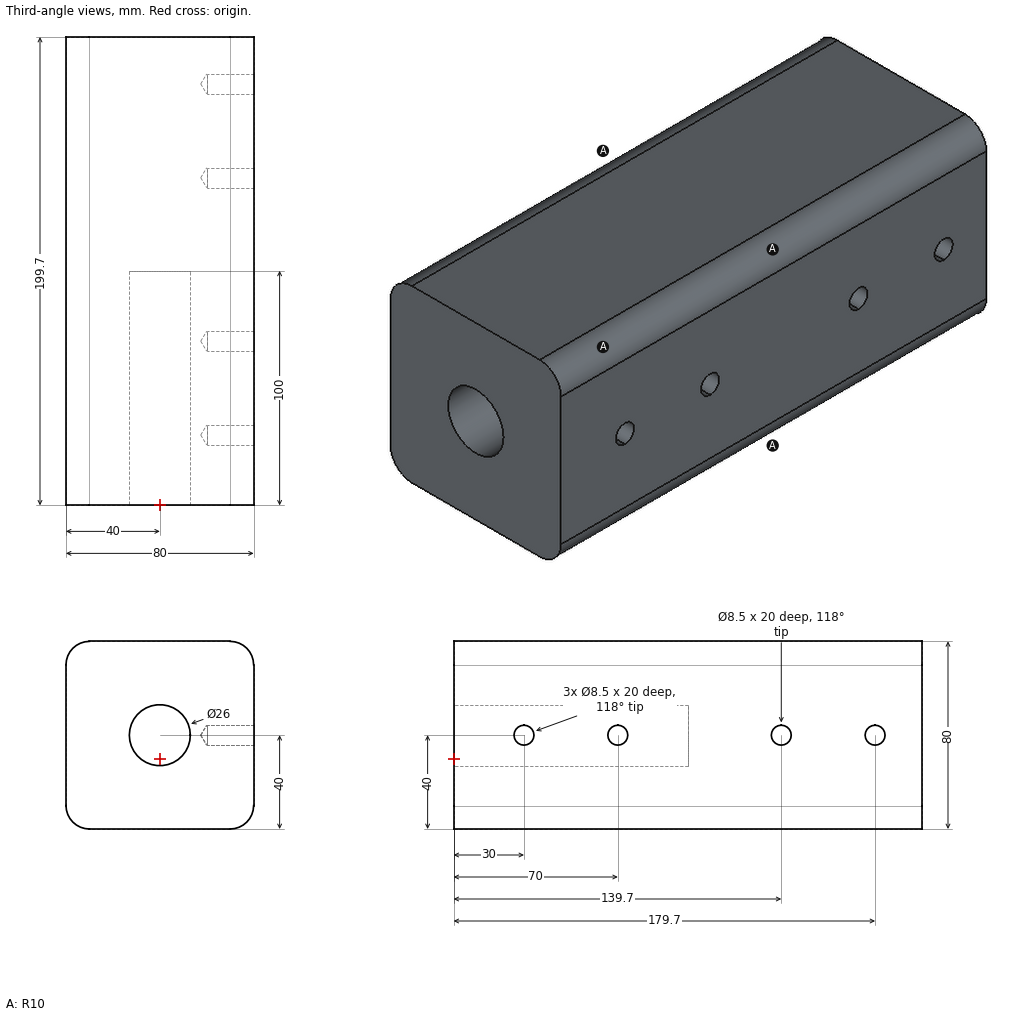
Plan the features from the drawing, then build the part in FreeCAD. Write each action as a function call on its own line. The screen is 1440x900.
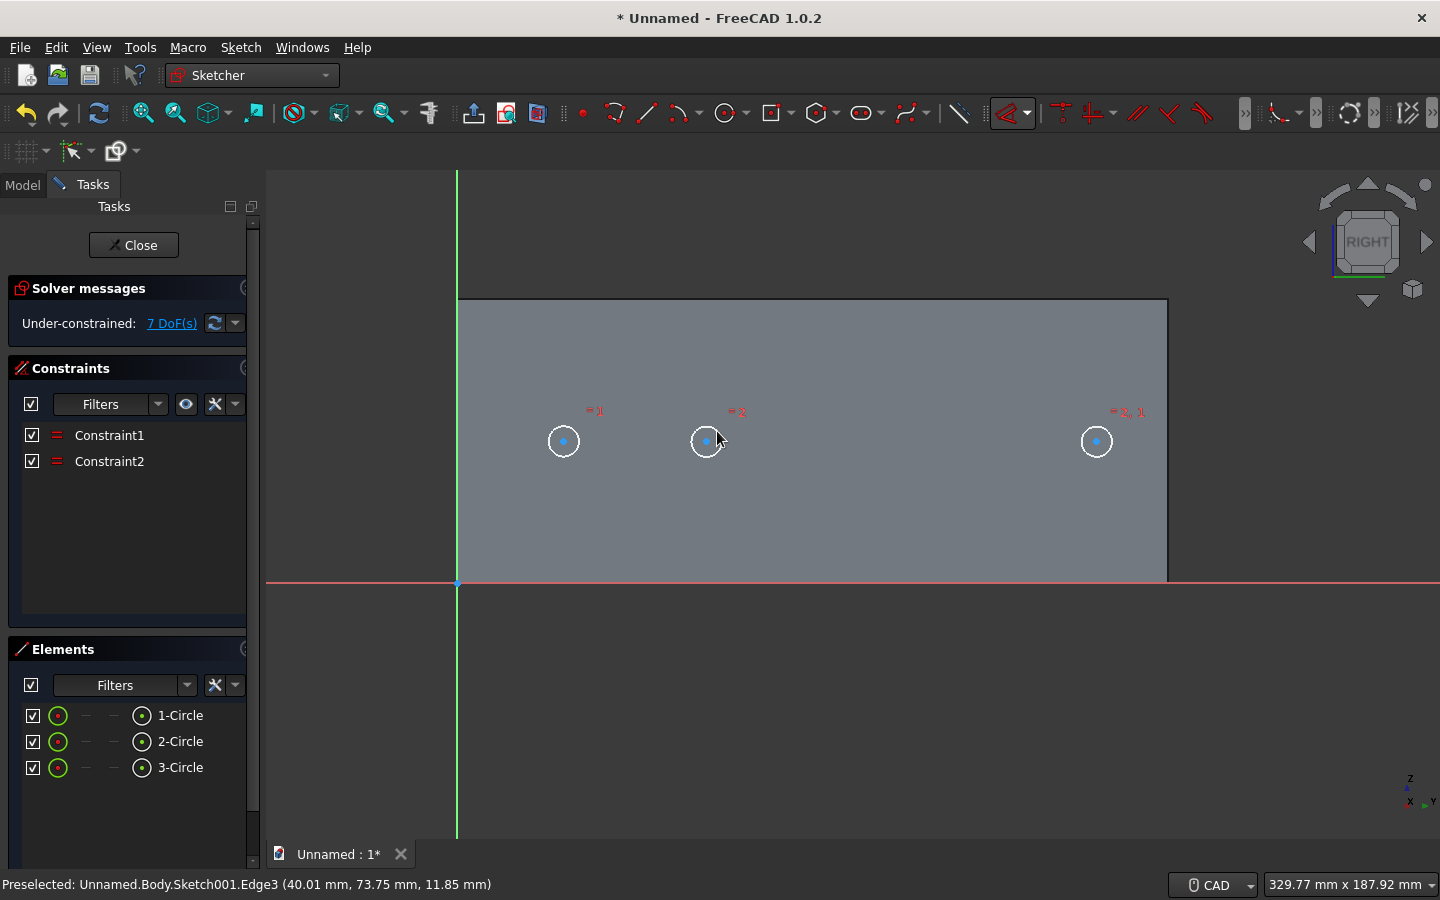
click(564, 441)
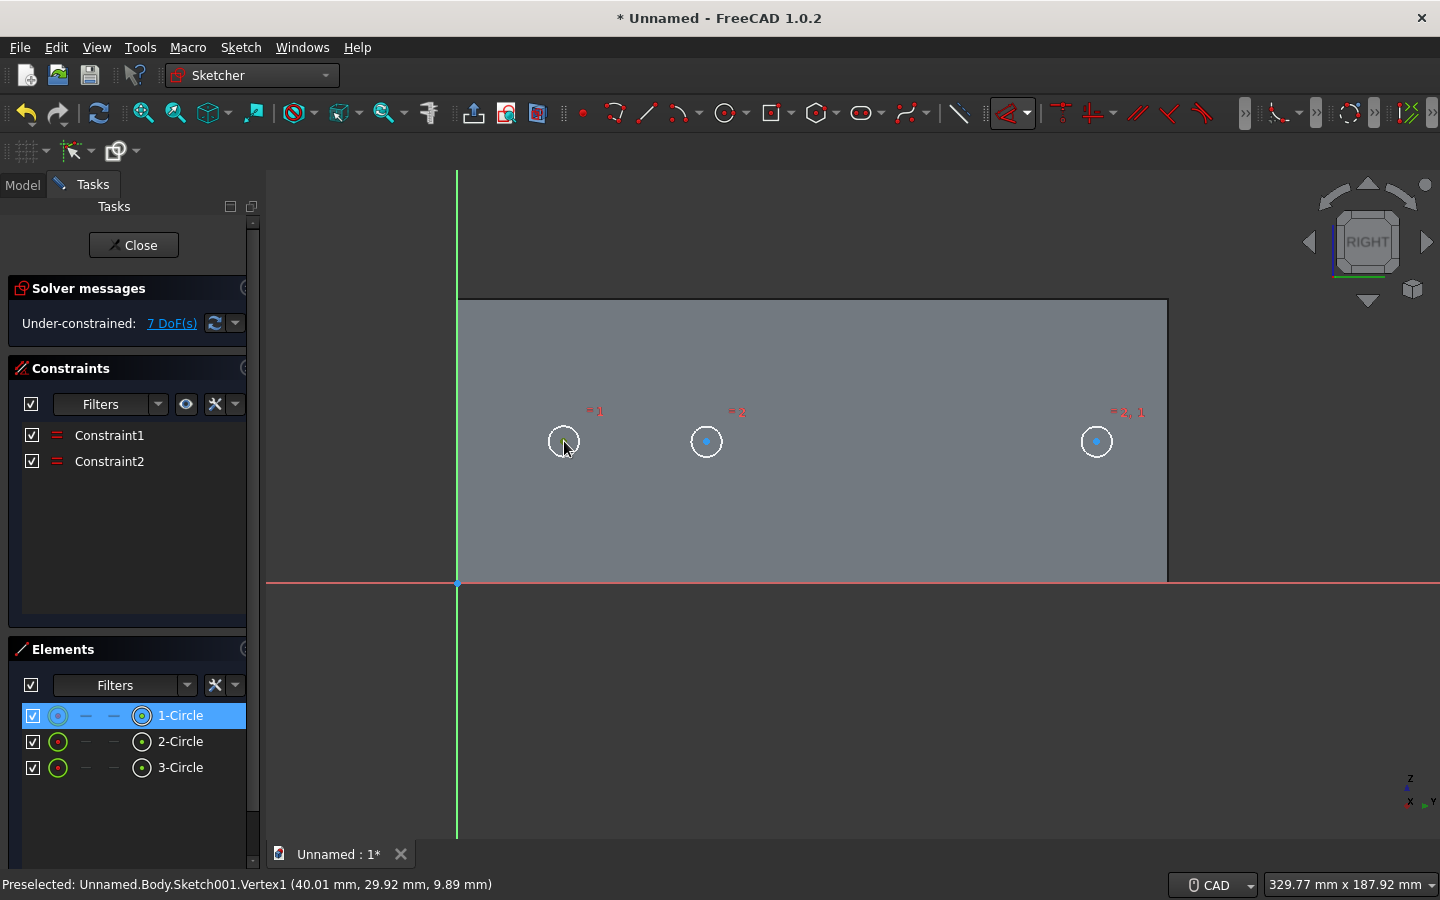
click(1097, 442)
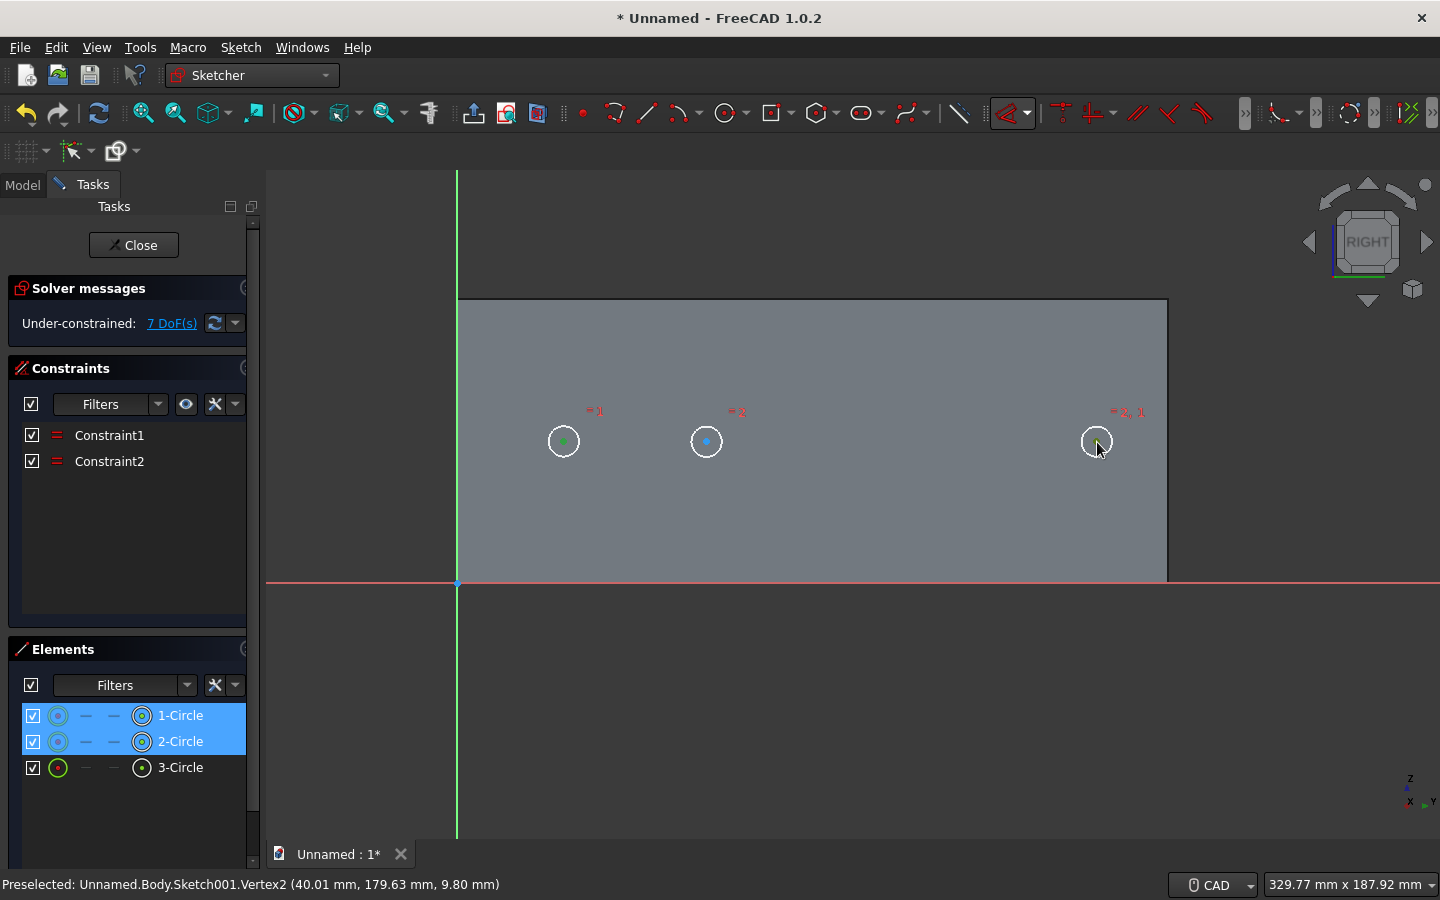
key(h)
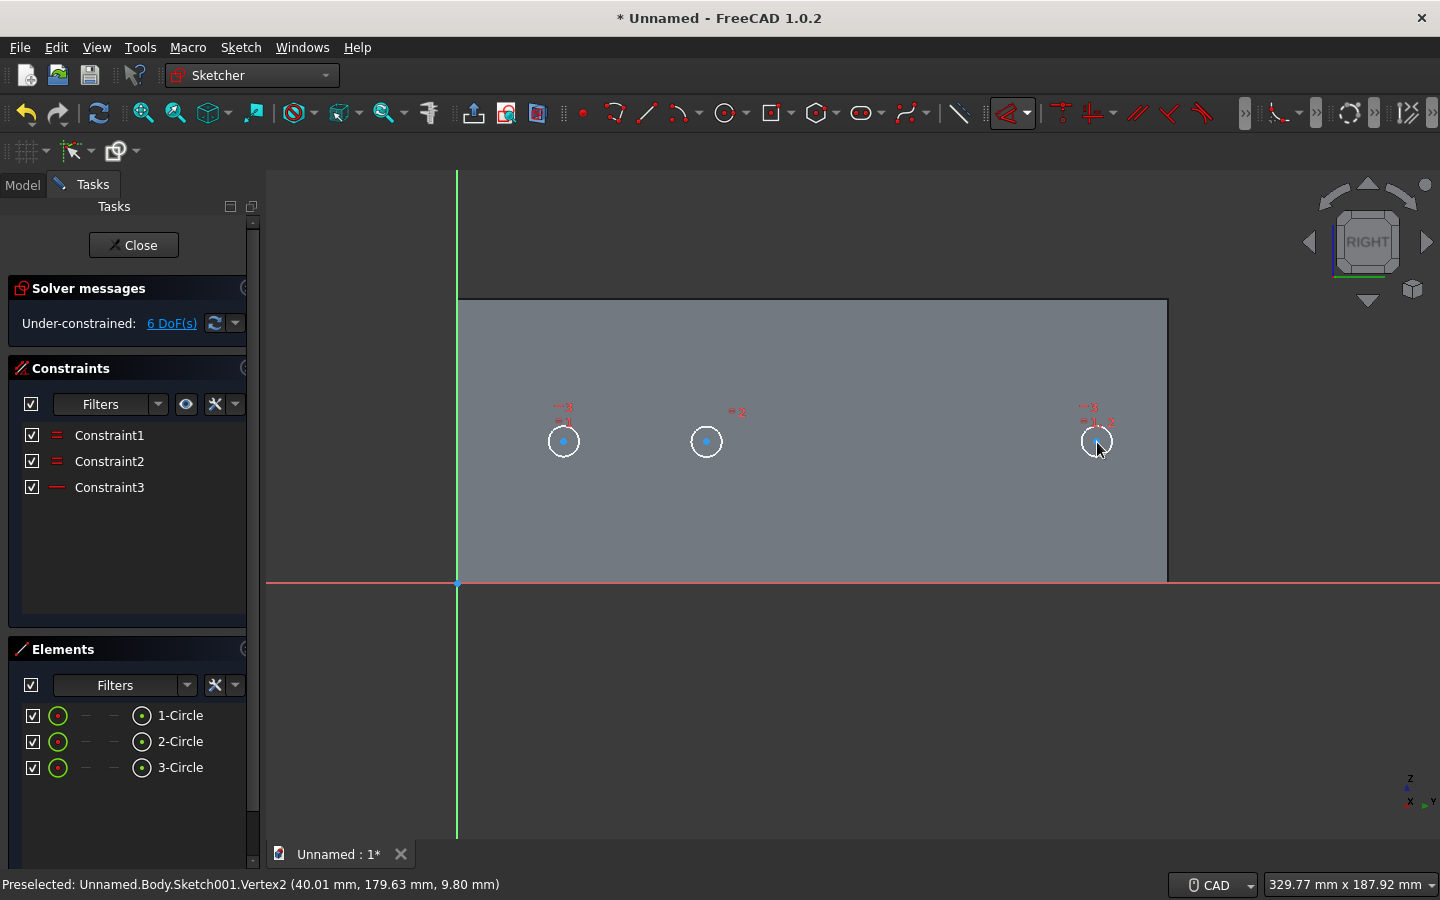
click(564, 441)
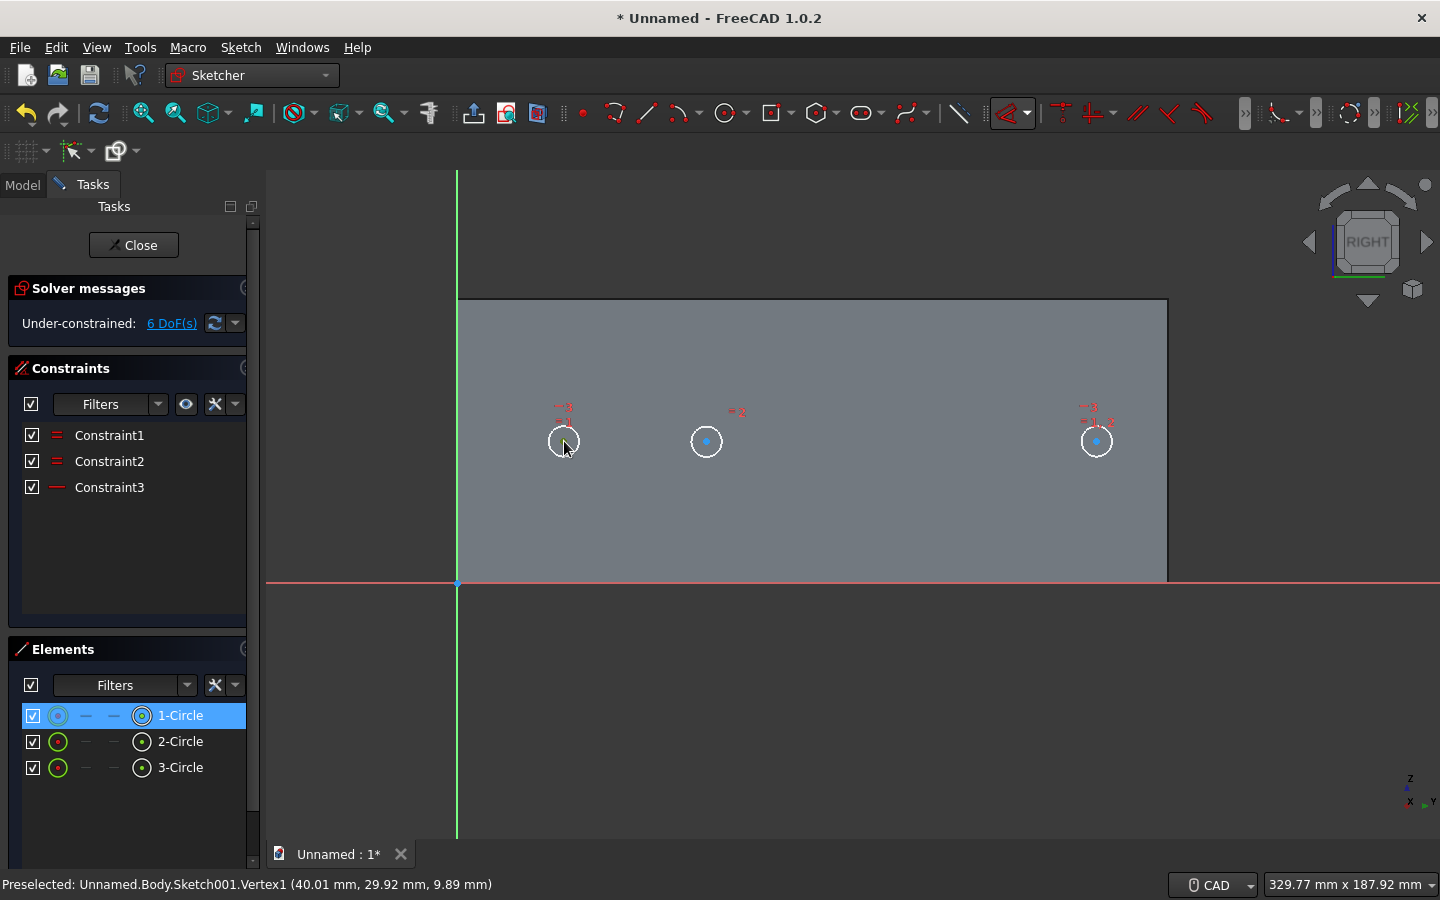
click(707, 442)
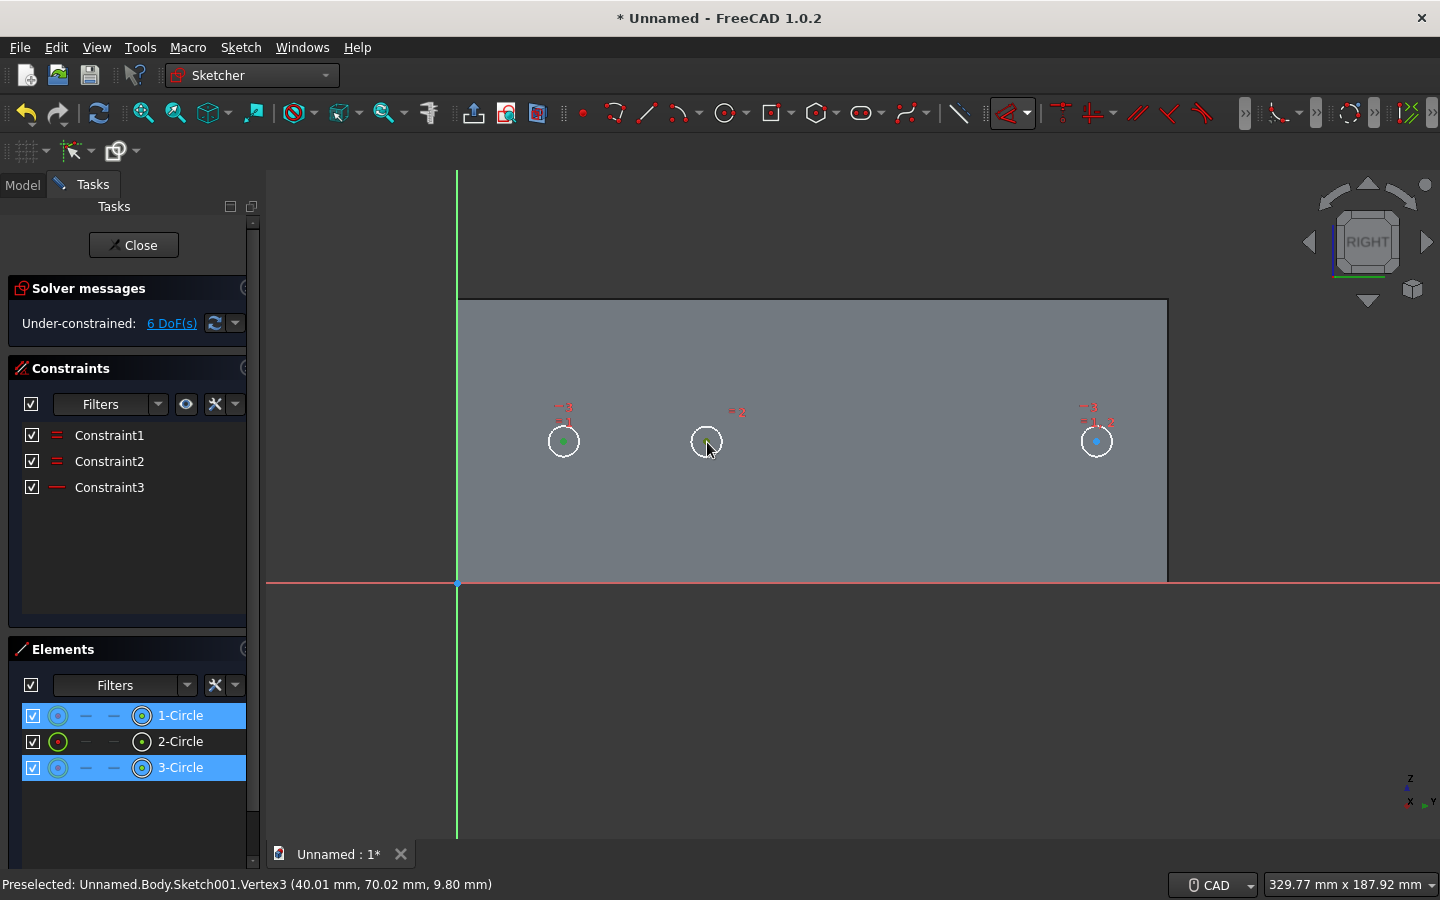
click(1116, 114)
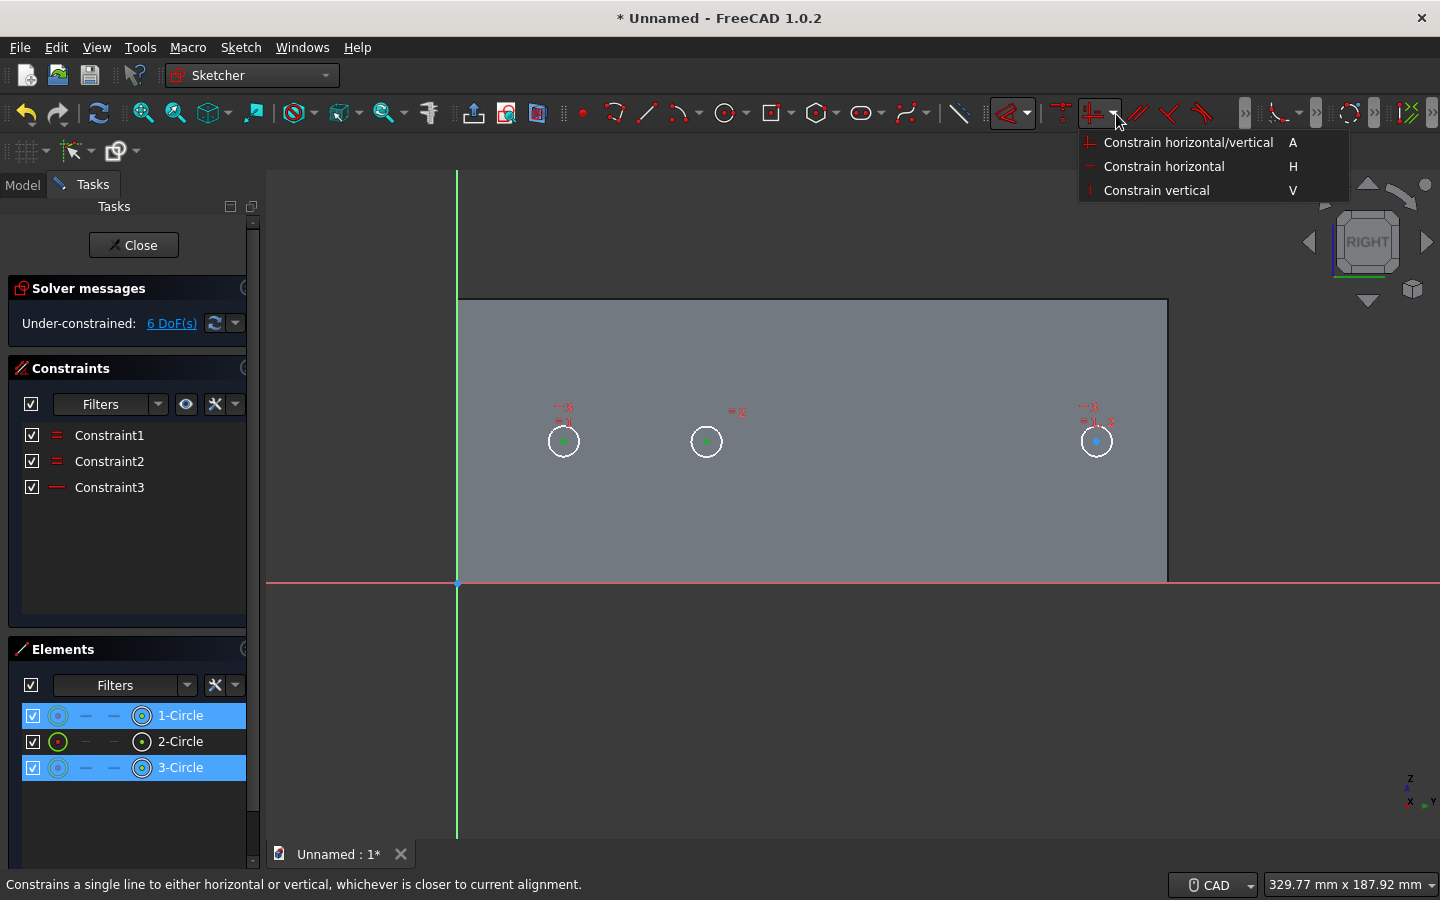
click(1214, 166)